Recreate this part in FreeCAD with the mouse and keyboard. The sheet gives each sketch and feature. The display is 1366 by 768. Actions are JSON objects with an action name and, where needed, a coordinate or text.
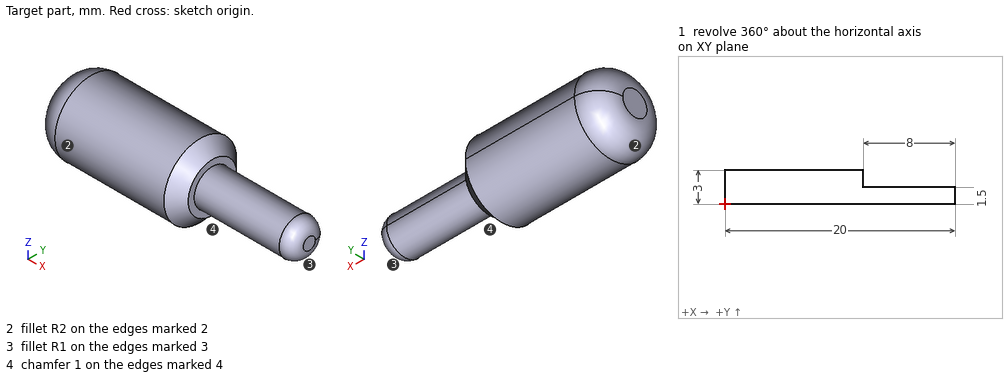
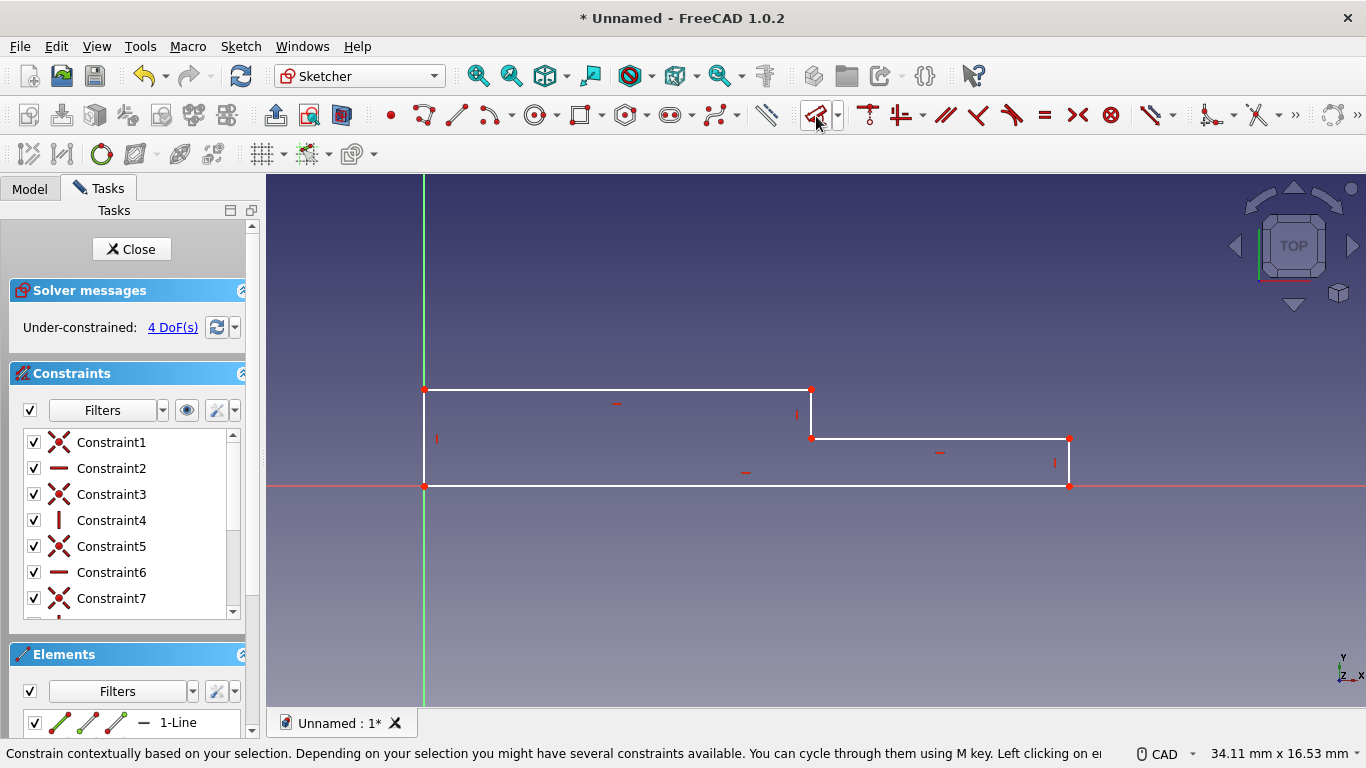
{"action": "left_click", "coordinate": [992, 439]}
{"action": "left_click", "coordinate": [940, 473]}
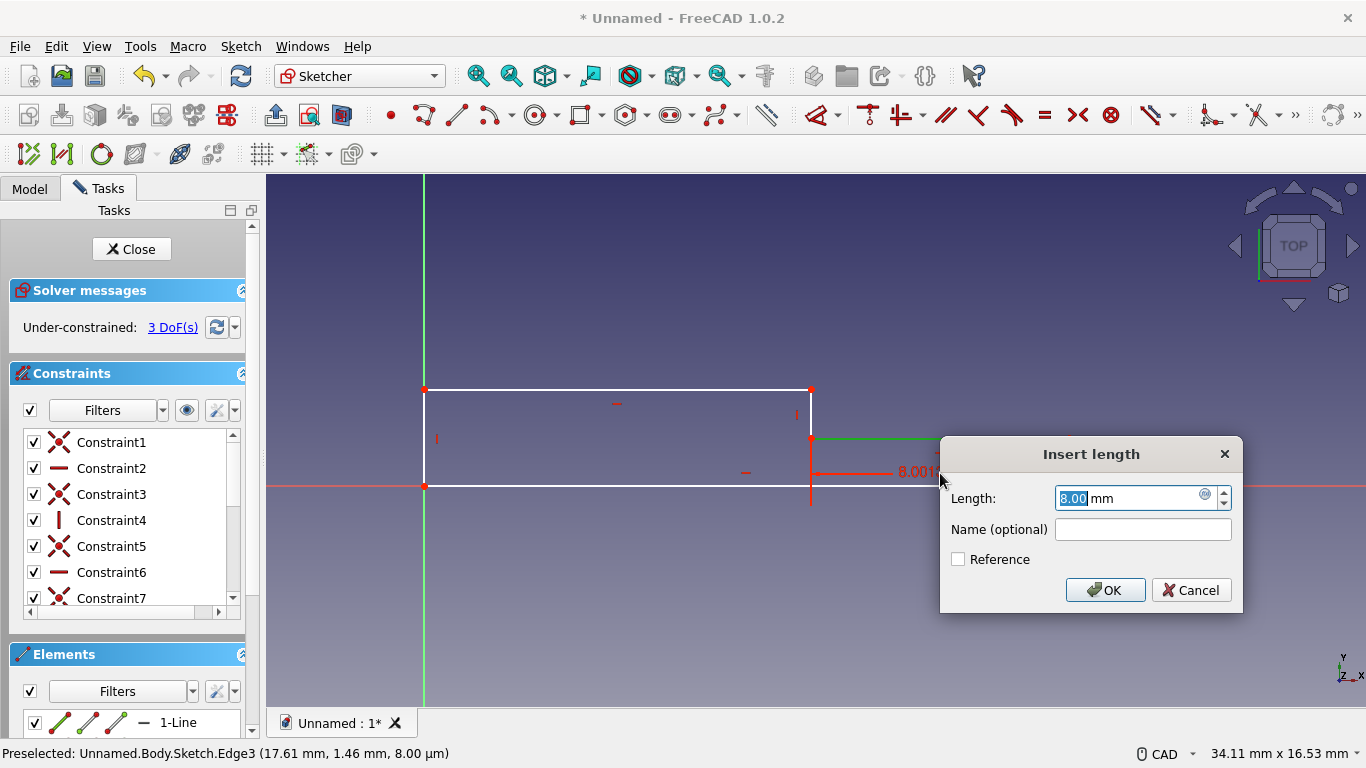
{"action": "type", "text": "8"}
{"action": "key", "text": "Return"}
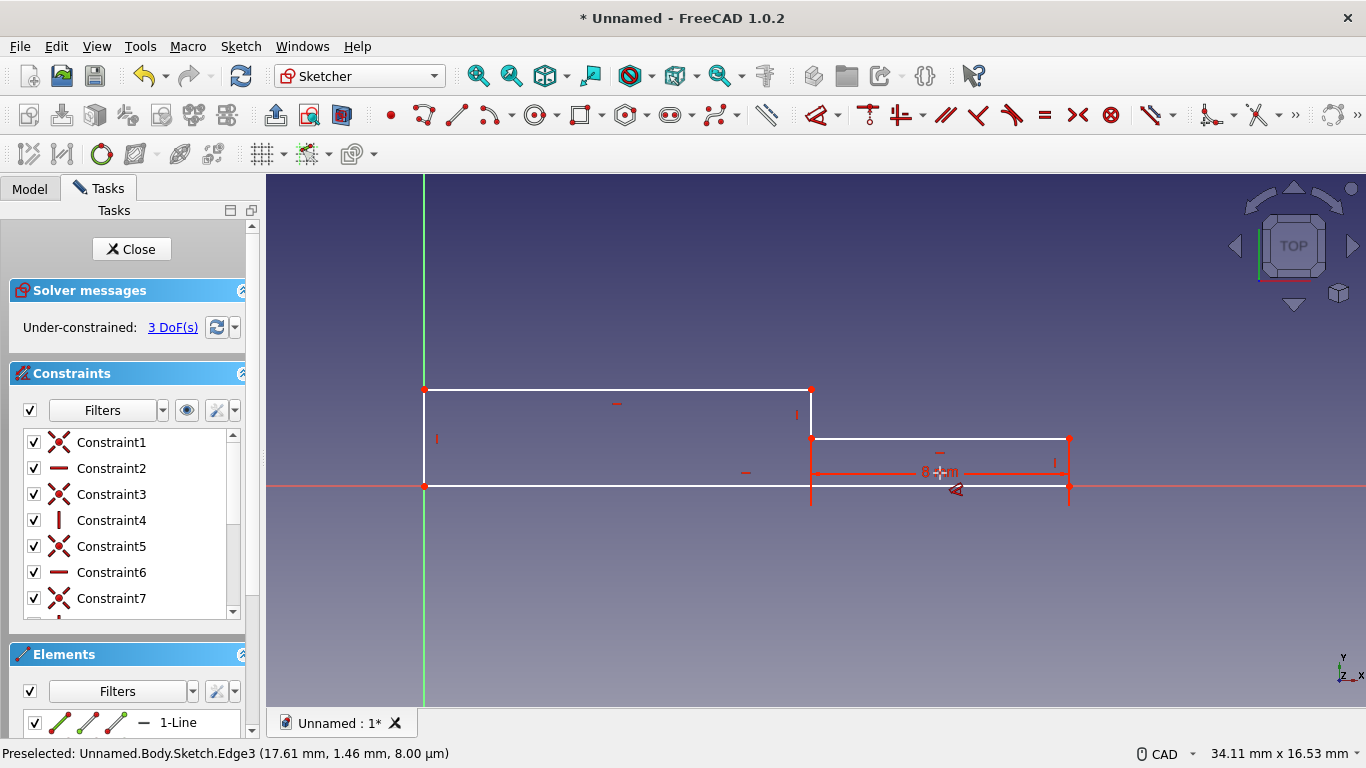
{"action": "left_click", "coordinate": [424, 419]}
{"action": "left_click", "coordinate": [390, 438]}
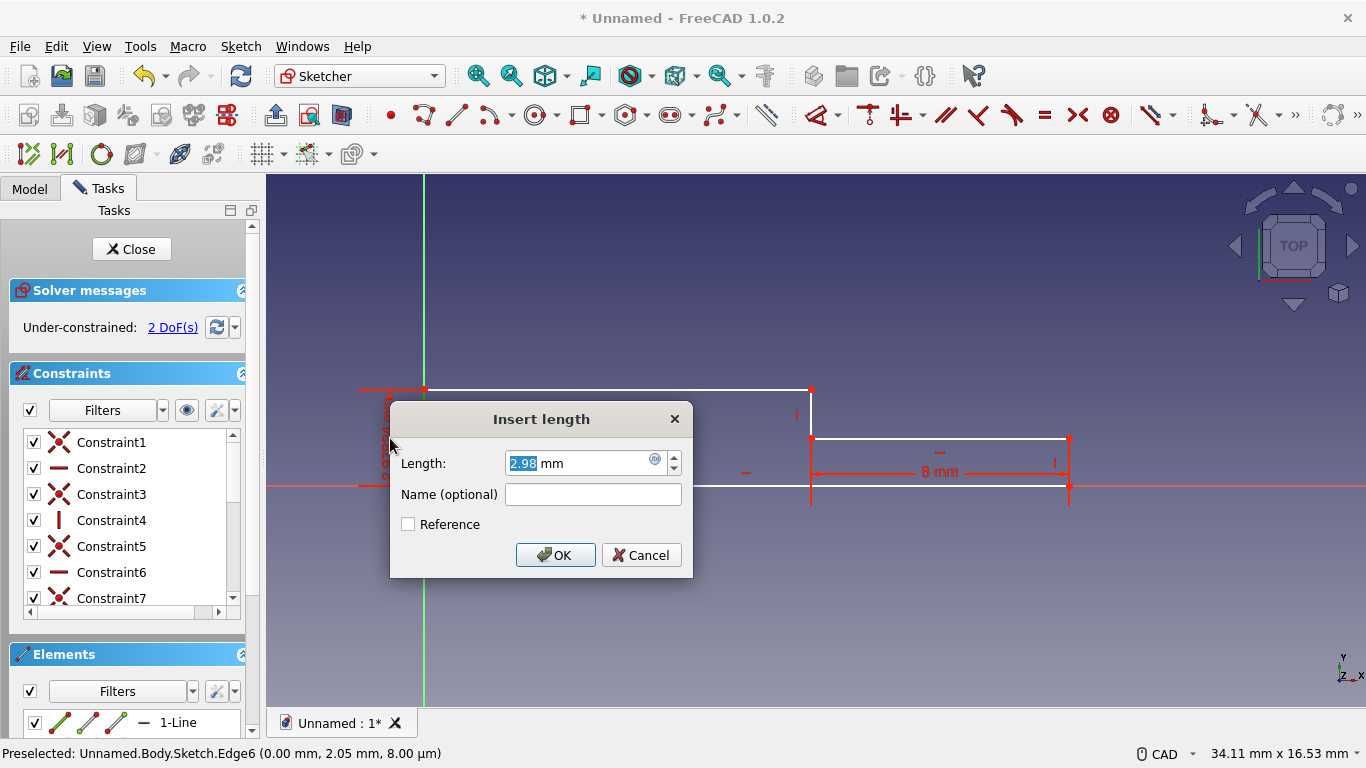
{"action": "type", "text": "3"}
{"action": "key", "text": "Return"}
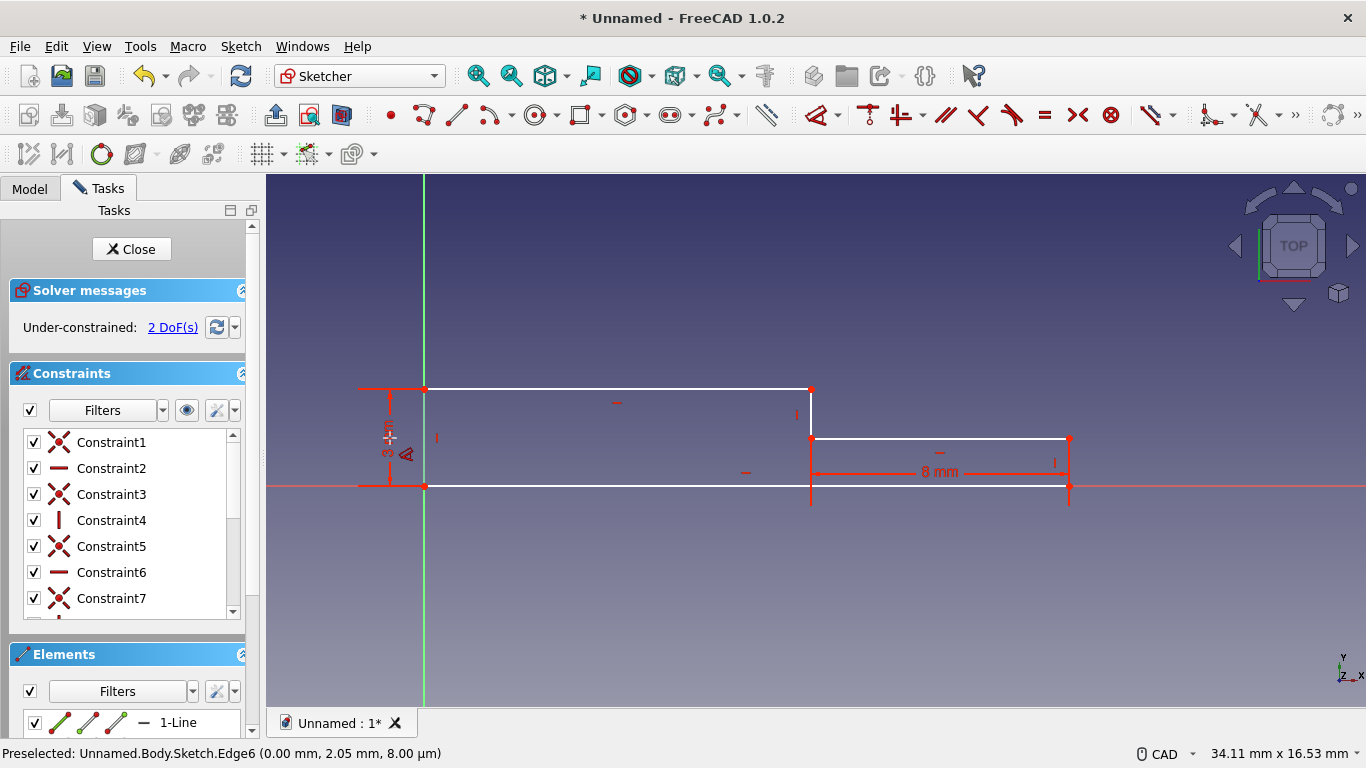
{"action": "left_click", "coordinate": [618, 486]}
{"action": "left_click", "coordinate": [747, 520]}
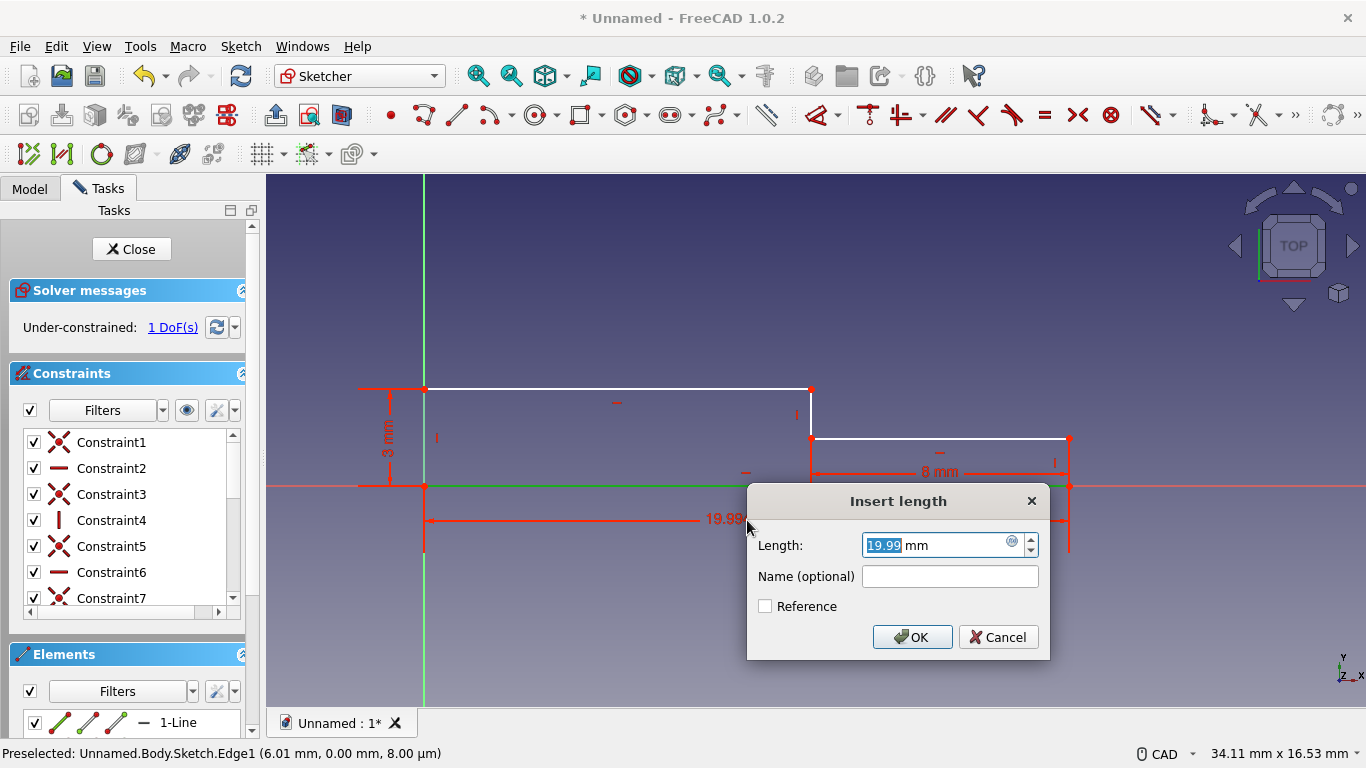
{"action": "type", "text": "20"}
{"action": "key", "text": "Return"}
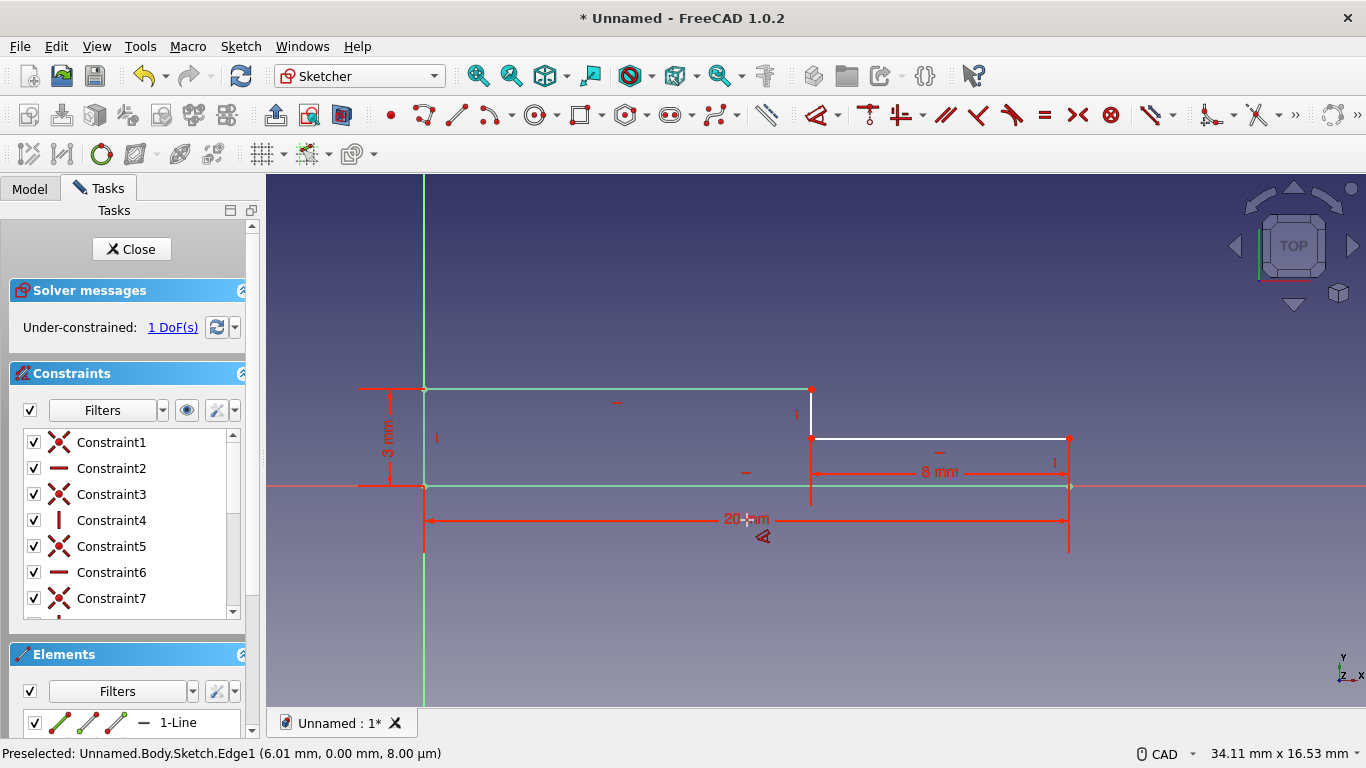
{"action": "left_click", "coordinate": [1069, 472]}
{"action": "left_click", "coordinate": [1103, 463]}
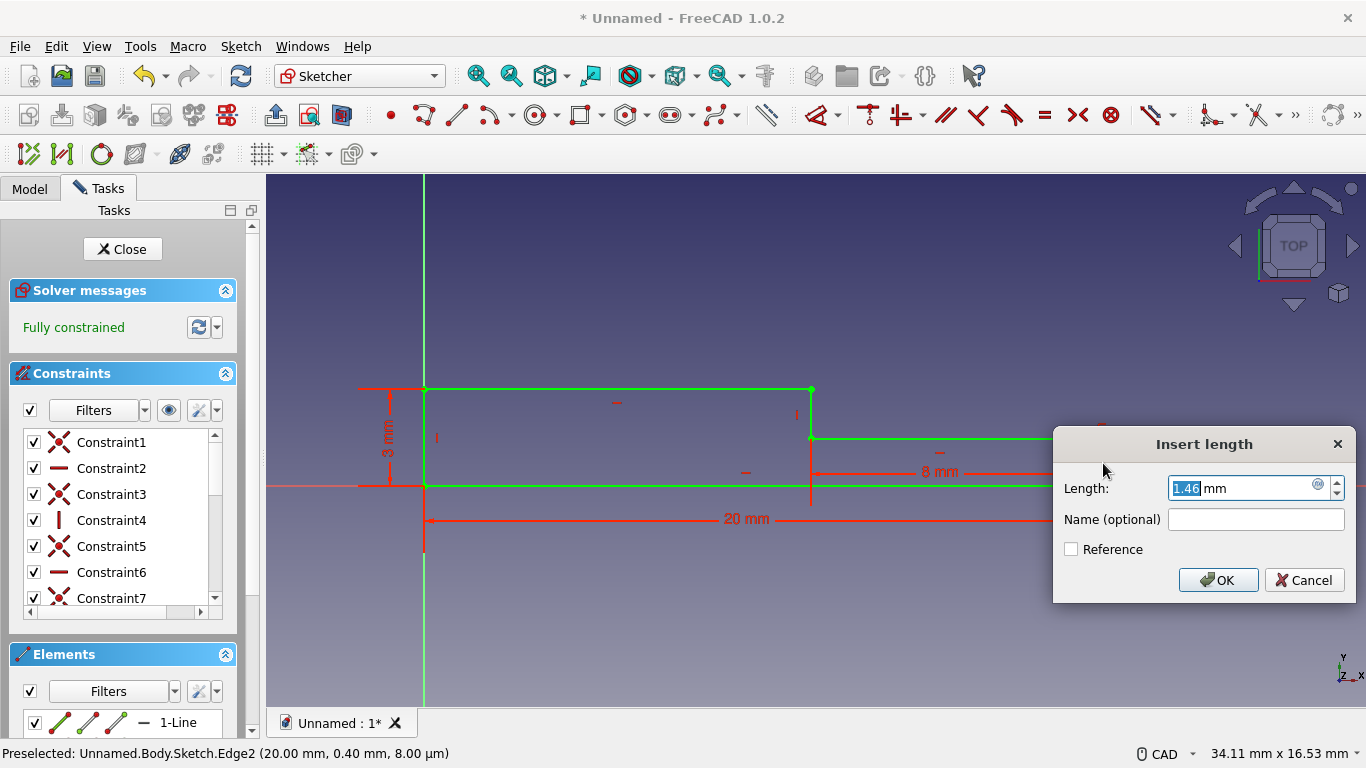
{"action": "type", "text": "1.5"}
{"action": "key", "text": "Return"}
{"action": "key", "text": "Escape"}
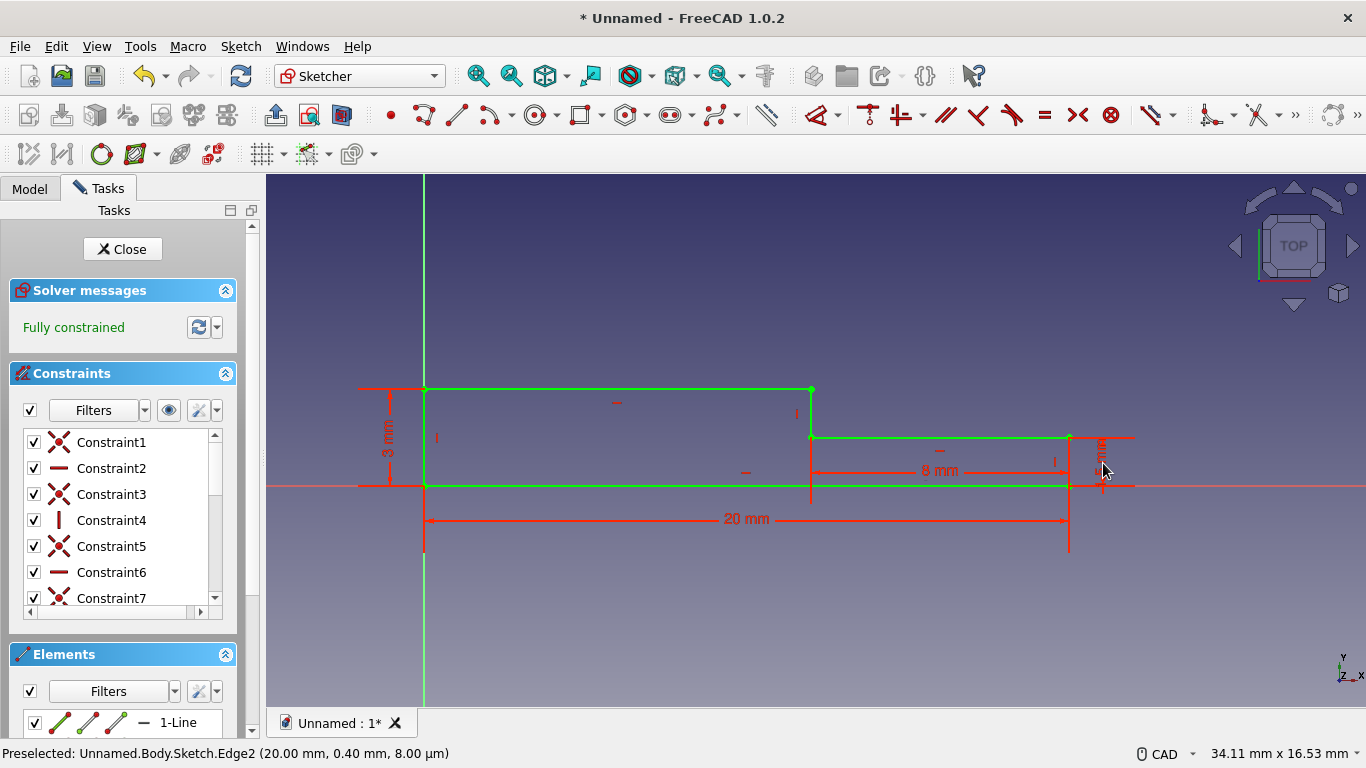
{"action": "left_click", "coordinate": [123, 249]}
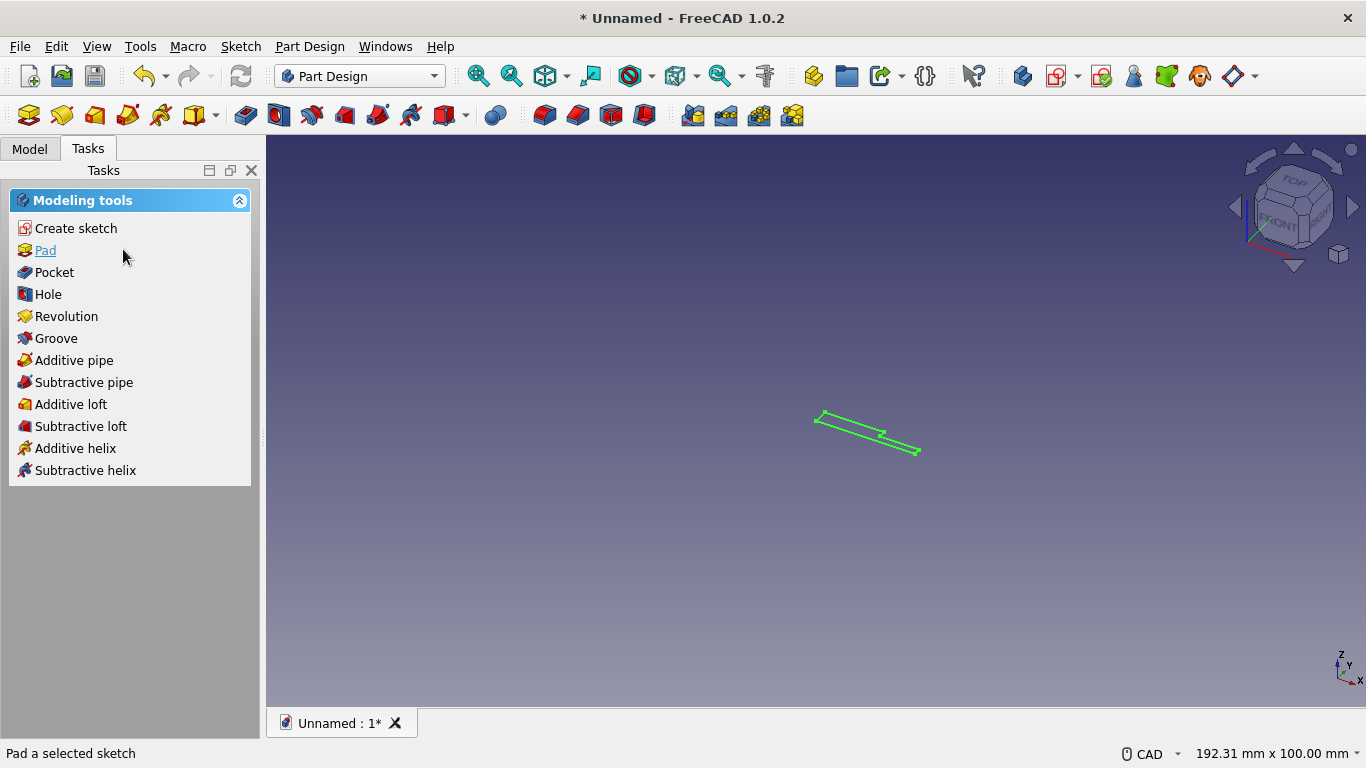
{"action": "left_click", "coordinate": [62, 116]}